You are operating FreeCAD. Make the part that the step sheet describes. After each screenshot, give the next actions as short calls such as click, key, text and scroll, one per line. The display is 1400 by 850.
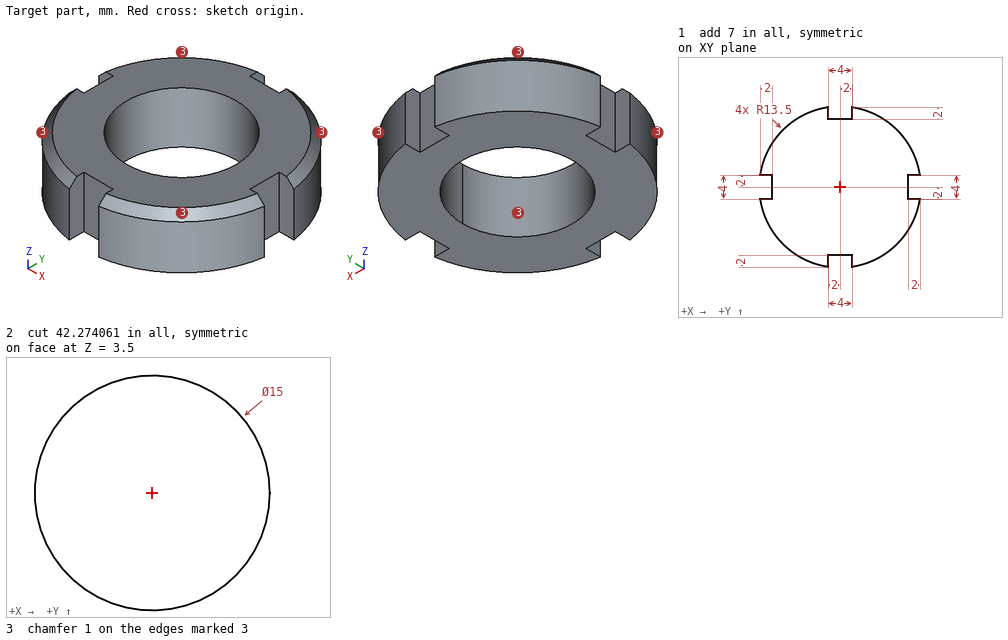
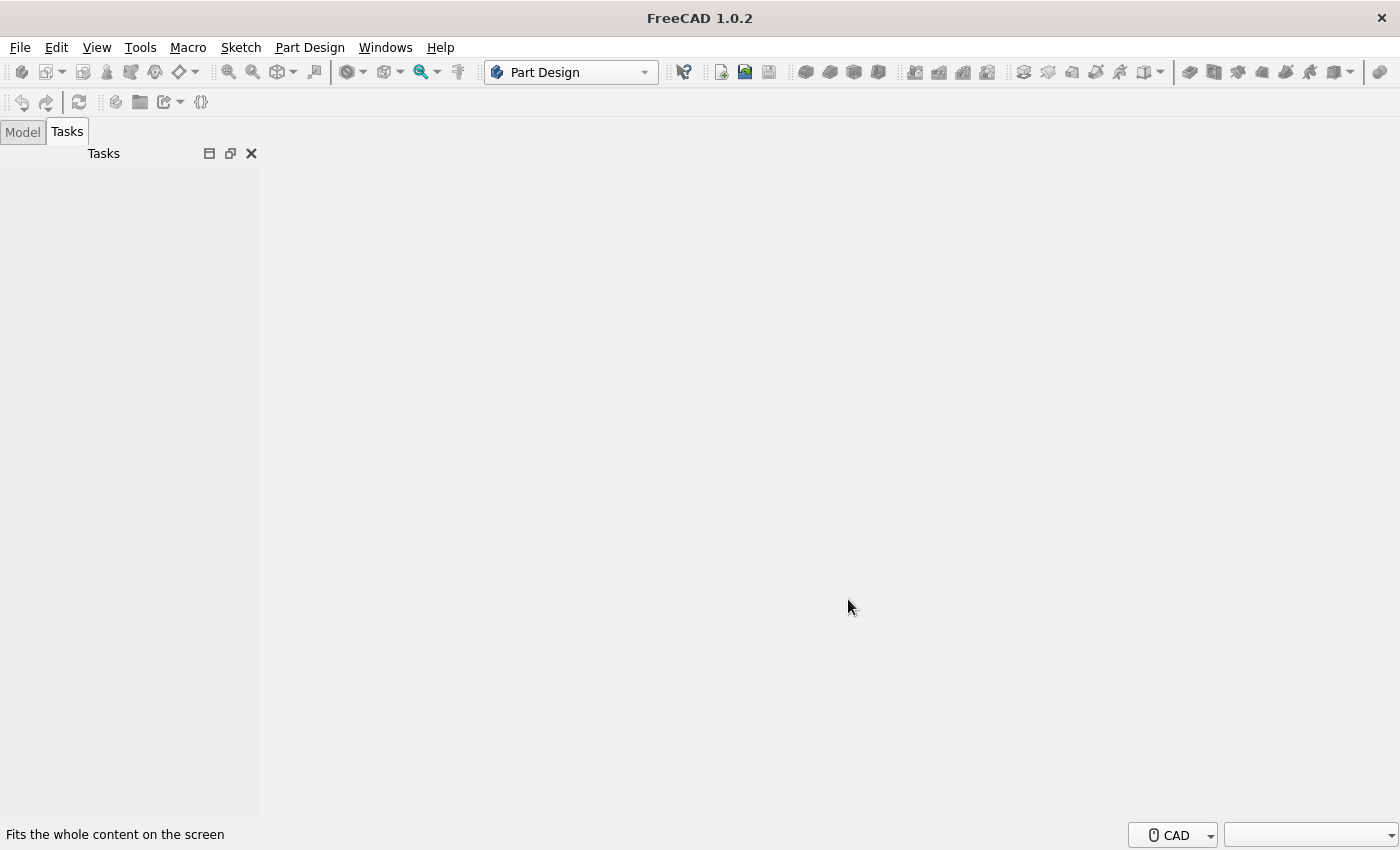
click(722, 72)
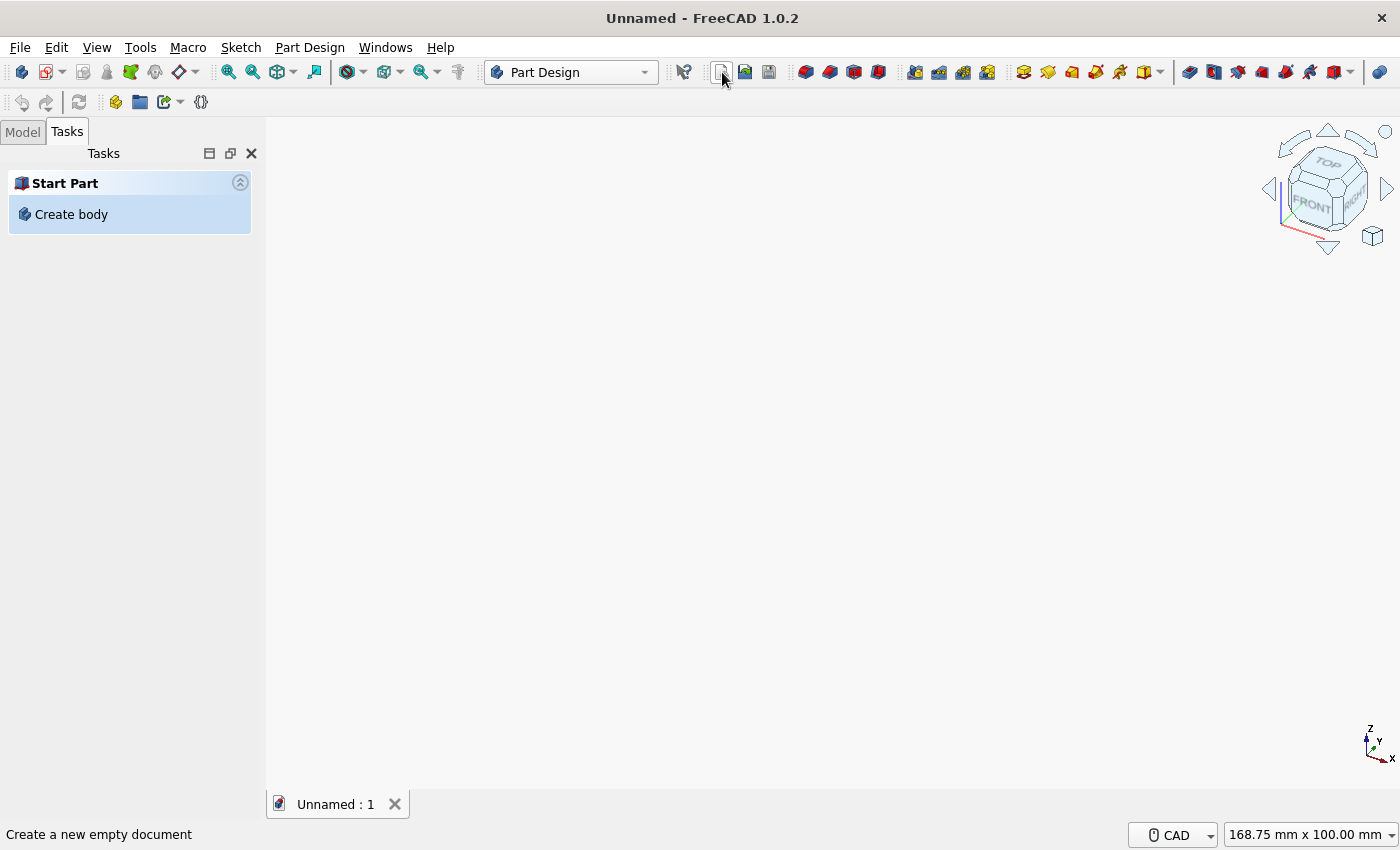
click(46, 72)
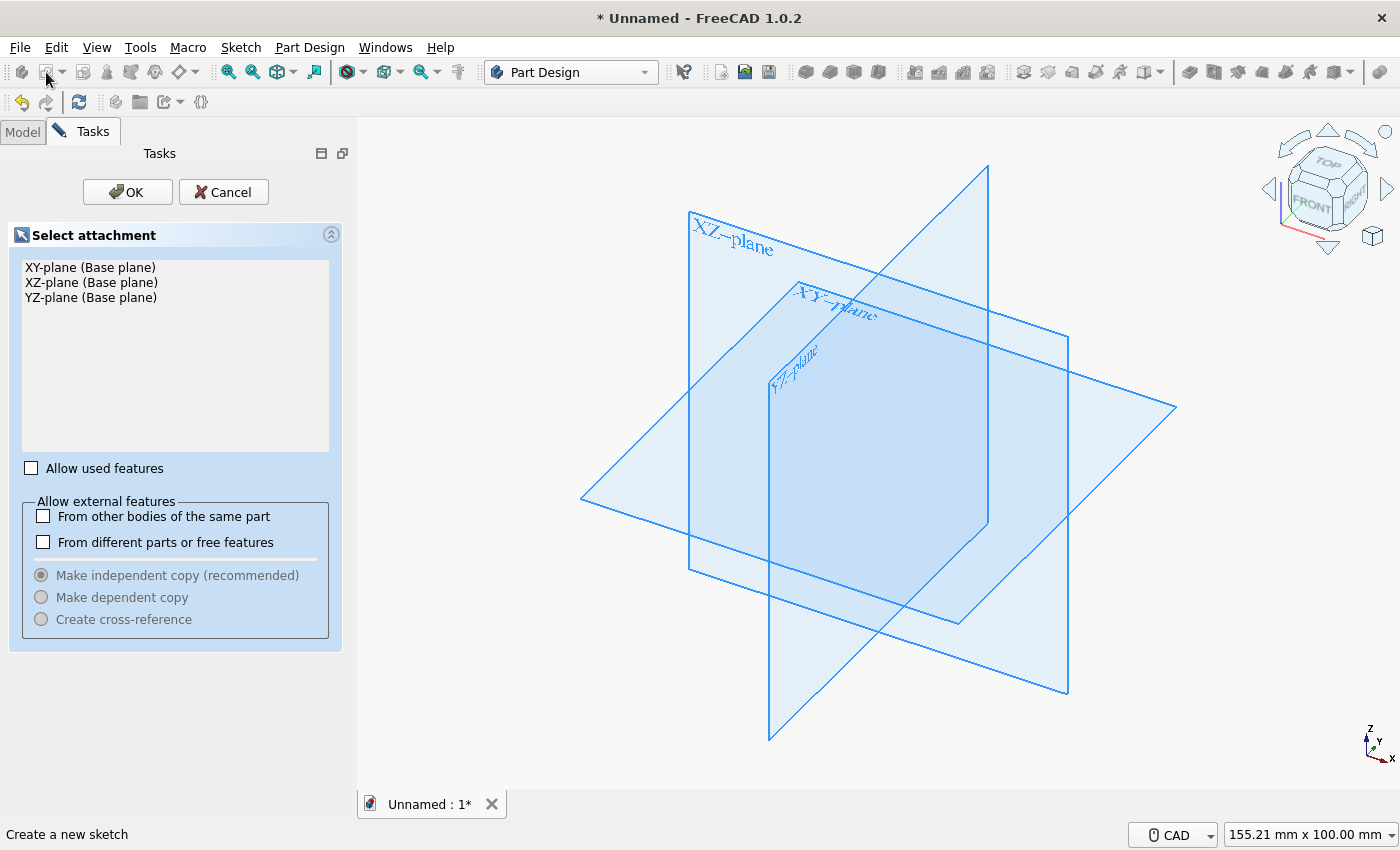
click(82, 268)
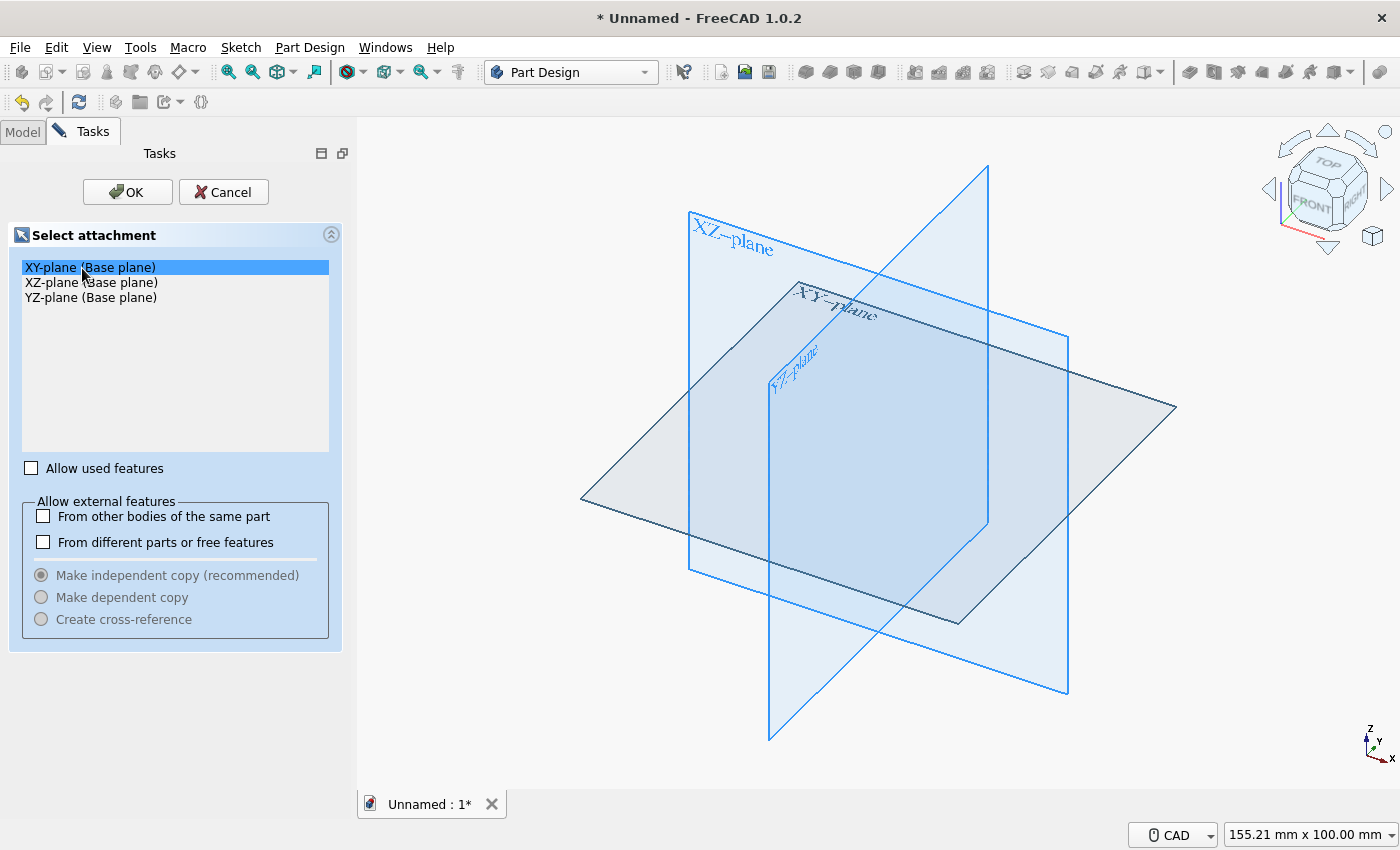
click(128, 192)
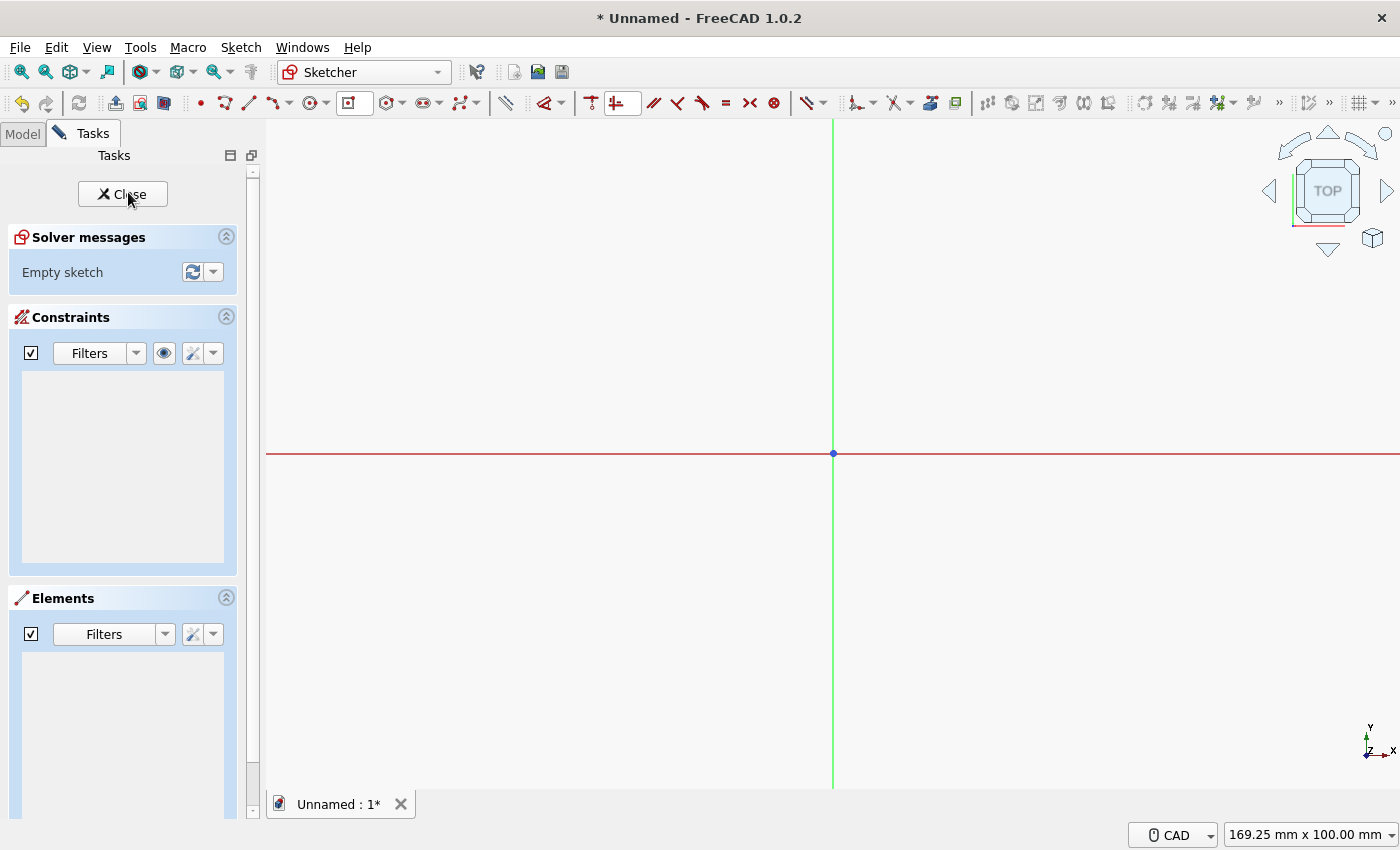
scroll(889, 454, up, 4)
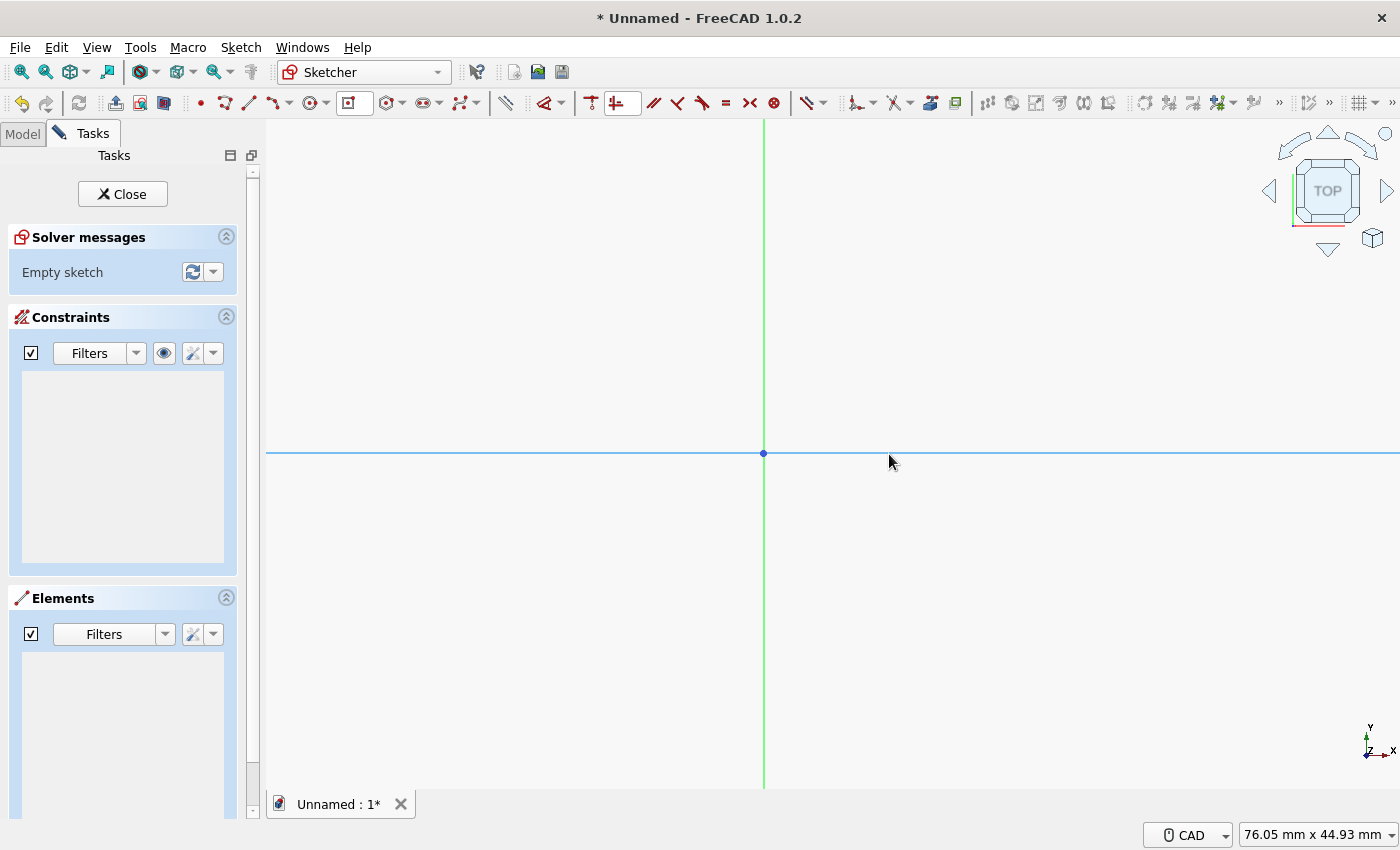
key(g)
key(m)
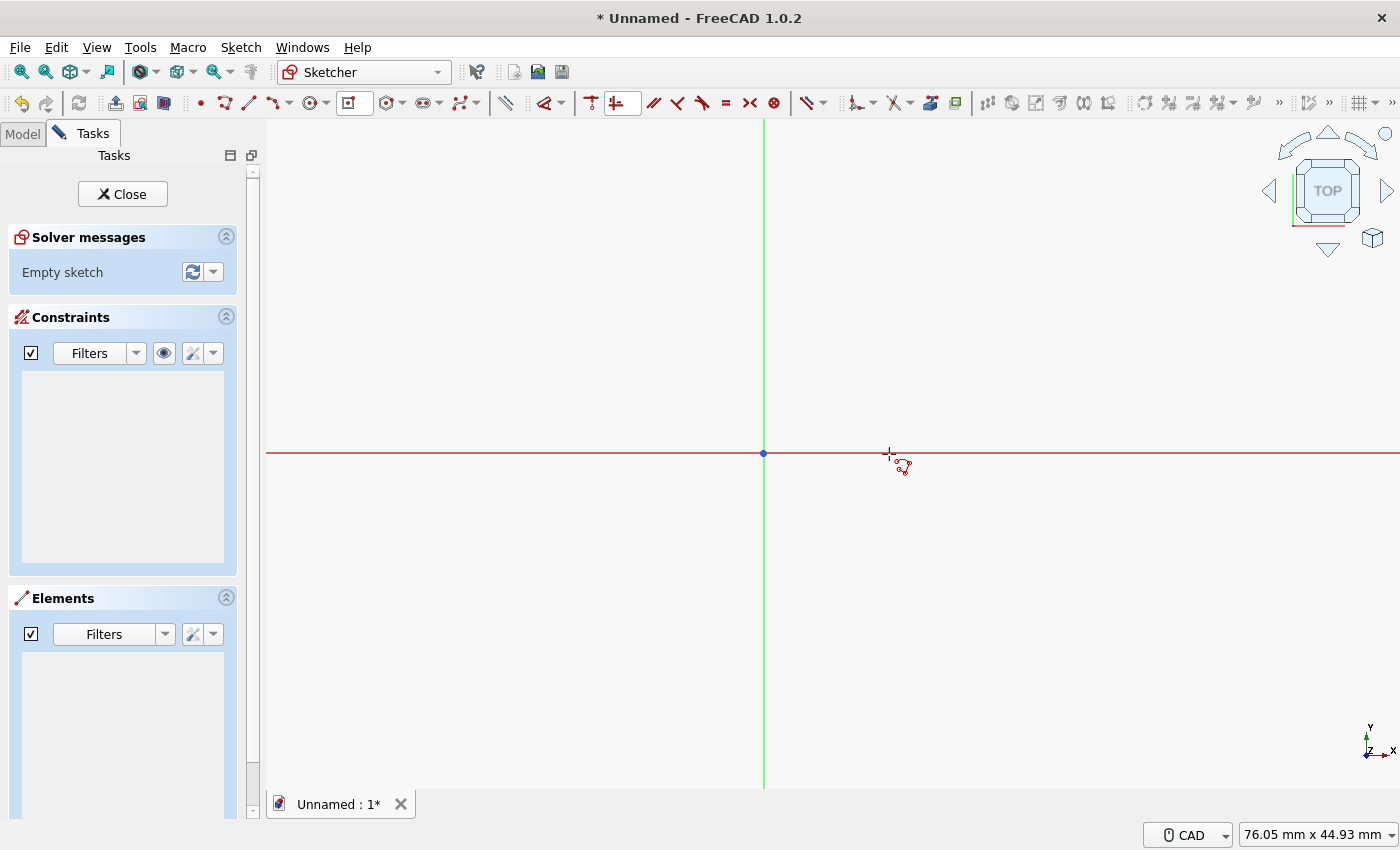
click(794, 254)
click(794, 284)
click(734, 284)
click(734, 254)
right_click(734, 254)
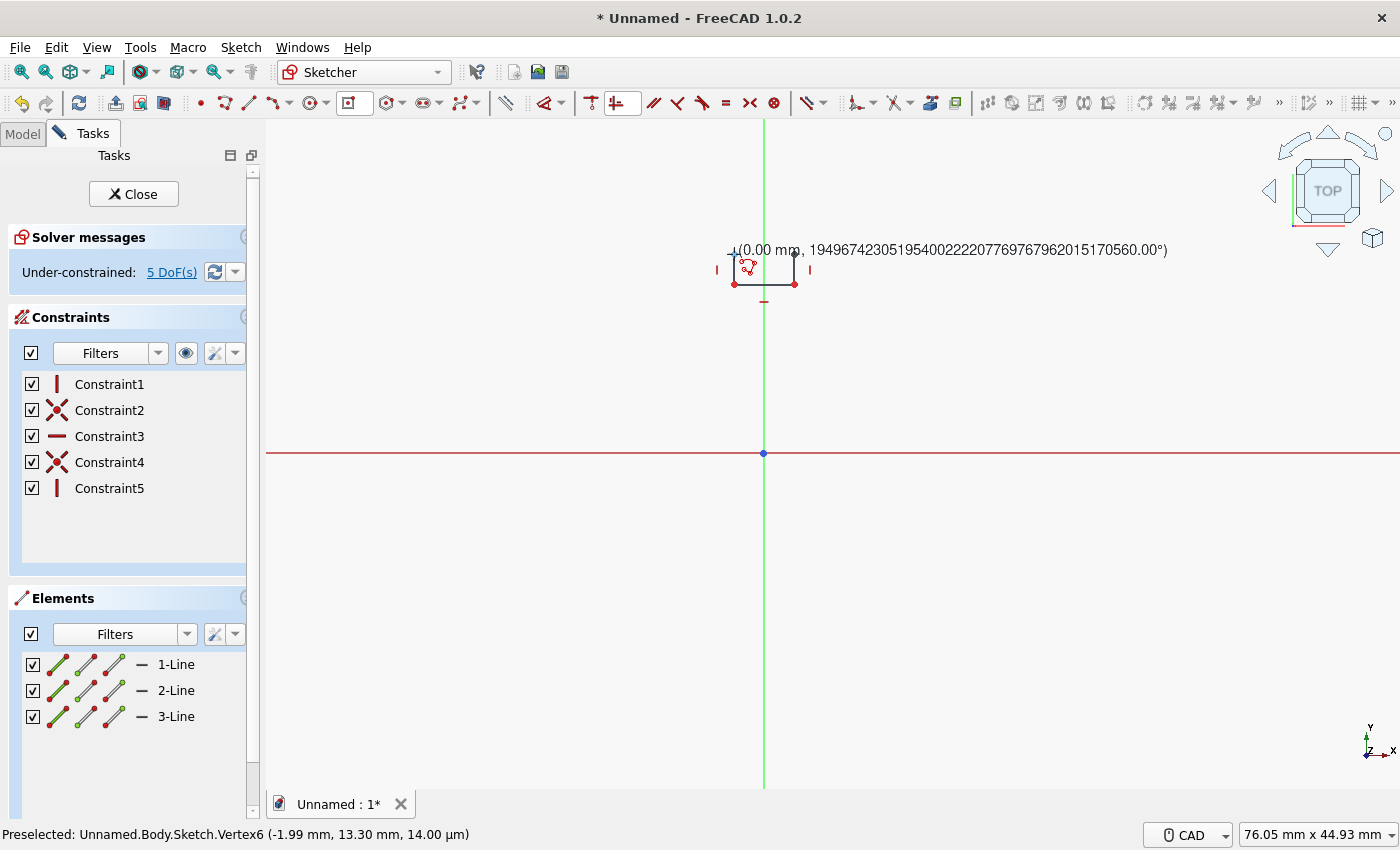
click(565, 424)
click(594, 424)
click(594, 483)
click(565, 483)
right_click(565, 483)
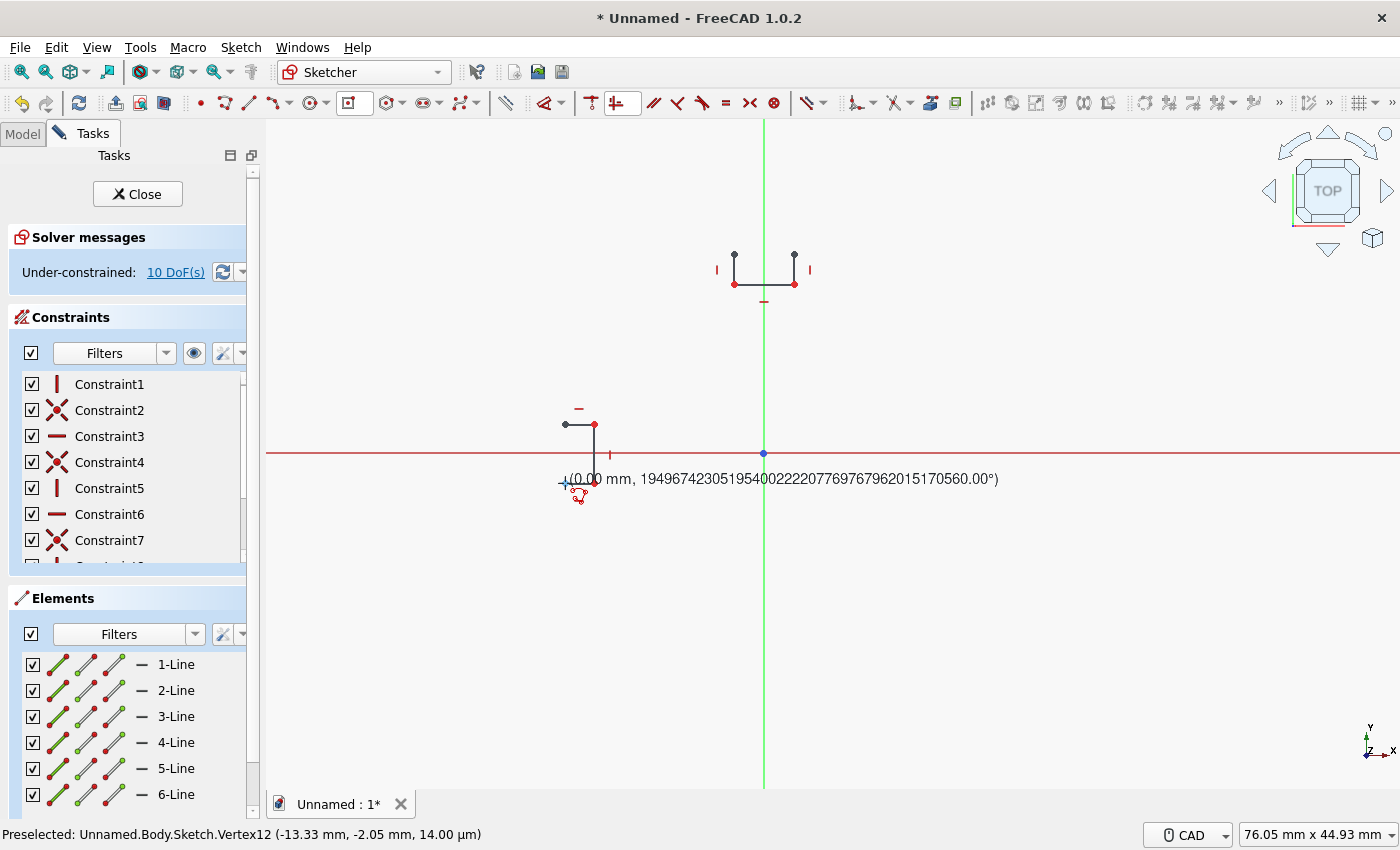
click(734, 652)
click(734, 623)
click(794, 623)
click(794, 652)
right_click(794, 652)